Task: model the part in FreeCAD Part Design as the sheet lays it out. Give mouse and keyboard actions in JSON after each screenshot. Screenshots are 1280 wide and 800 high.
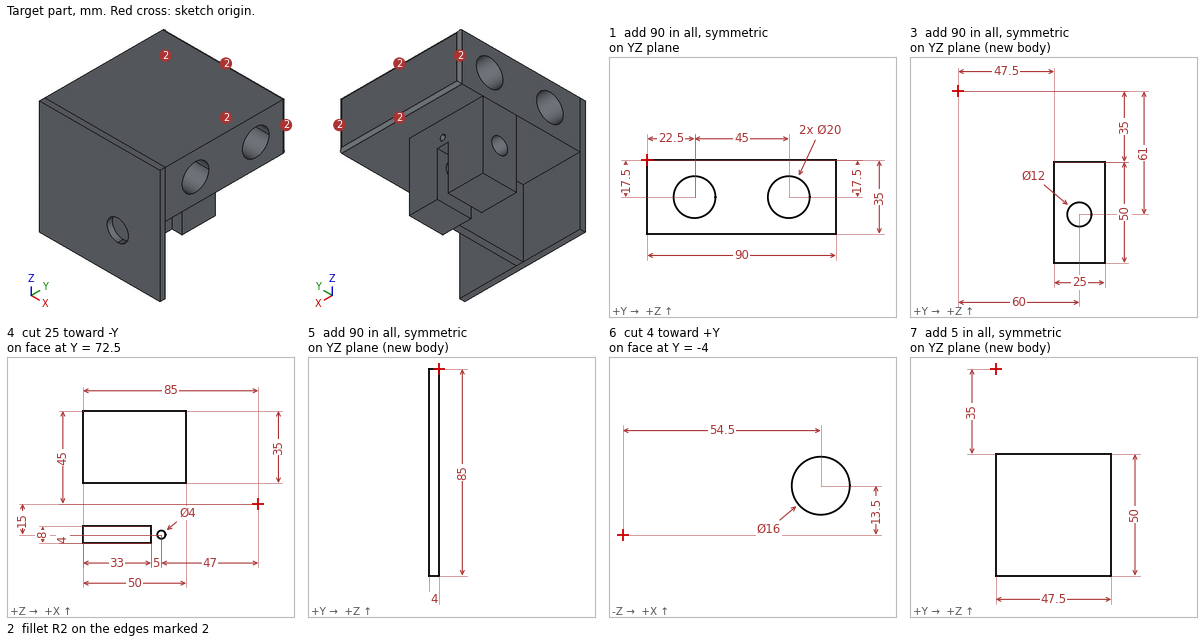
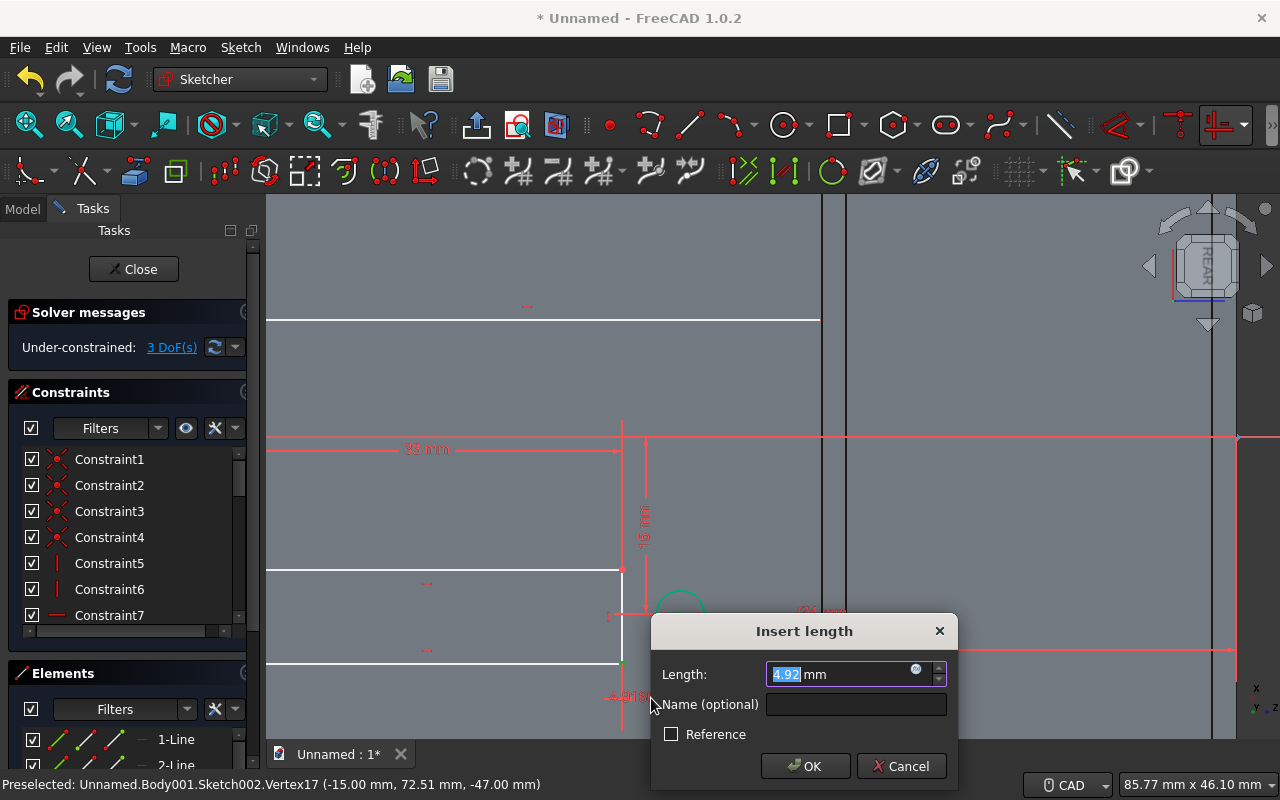
{"action": "type", "text": "5"}
{"action": "key", "text": "Return"}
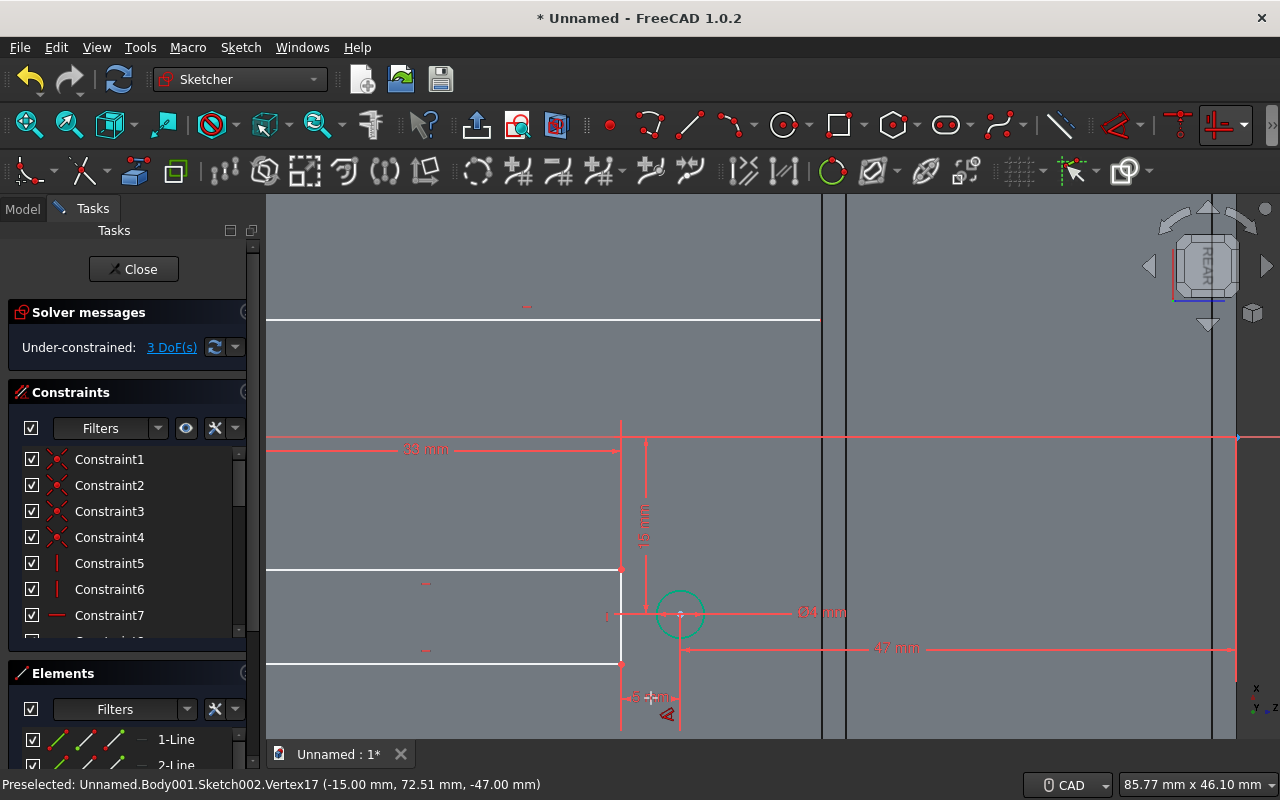
{"action": "left_click", "coordinate": [621, 664]}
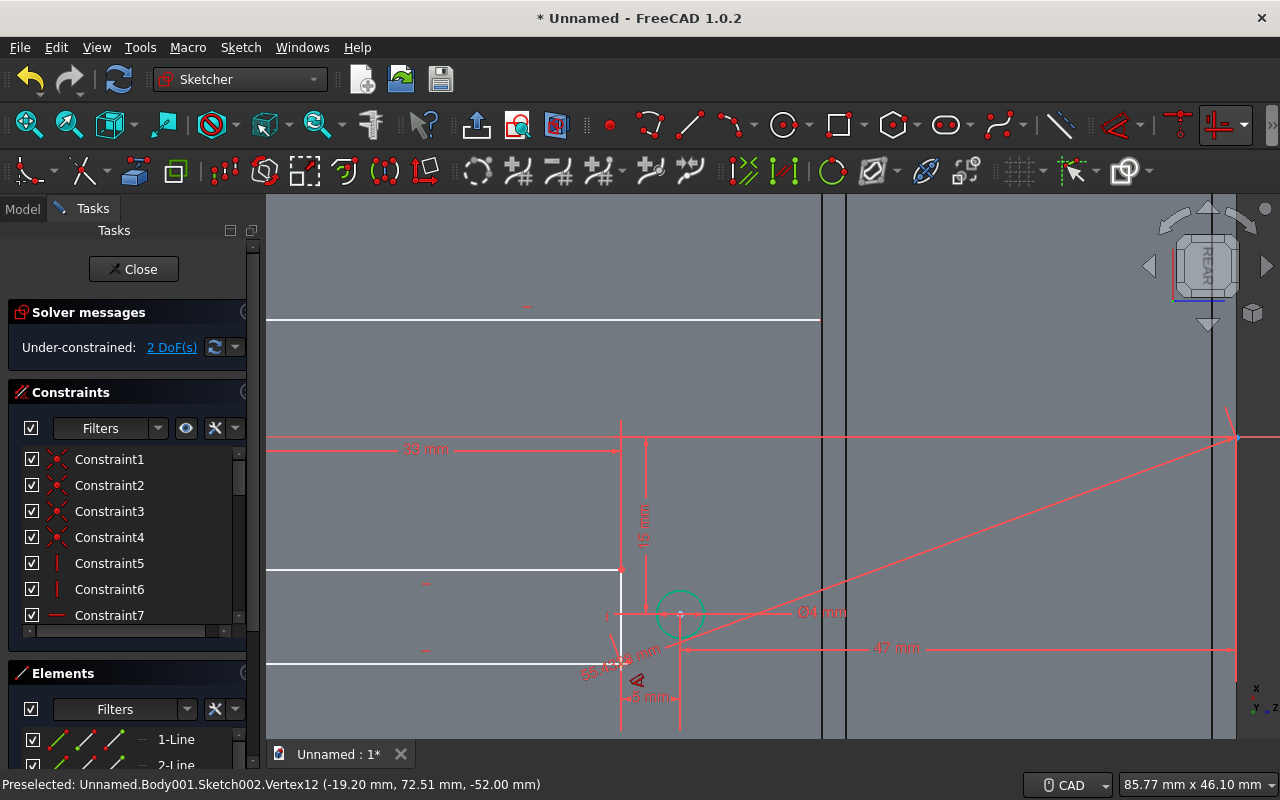
{"action": "left_click", "coordinate": [680, 614]}
{"action": "left_click", "coordinate": [587, 639]}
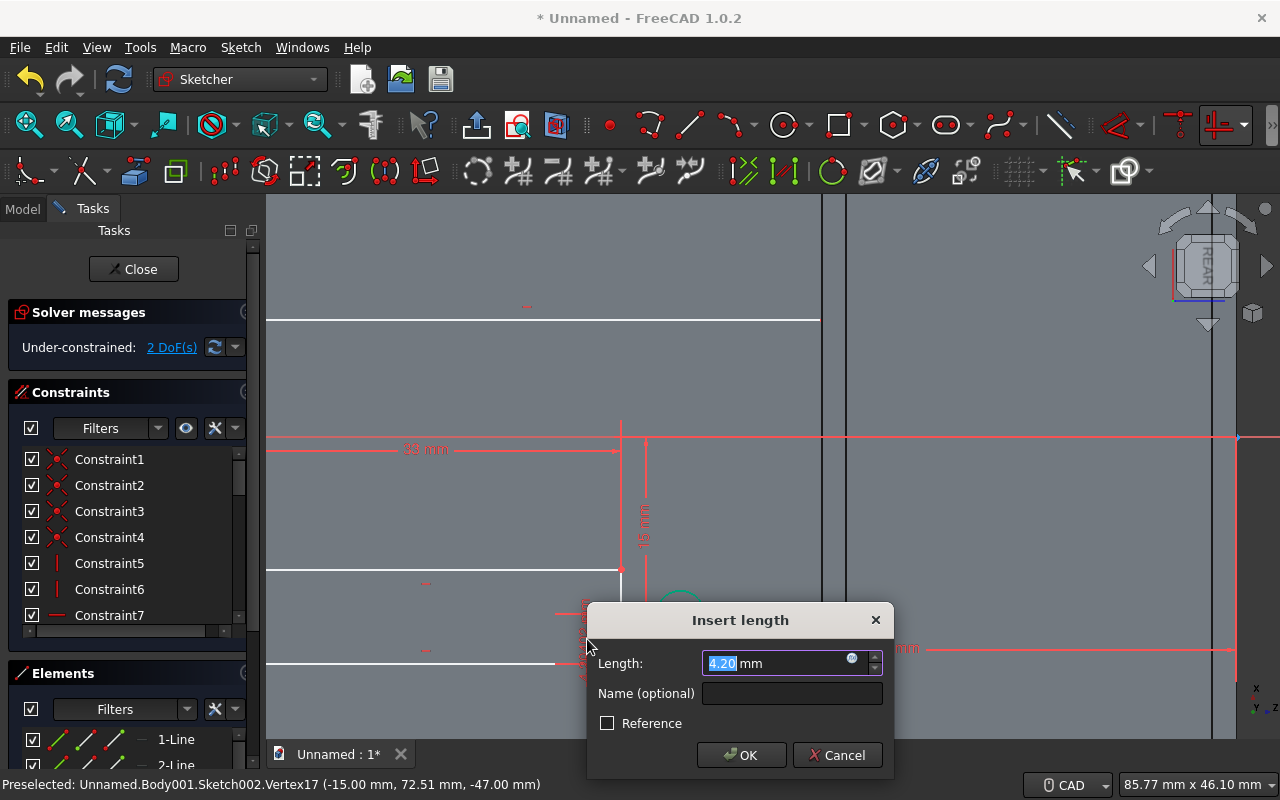
{"action": "type", "text": "4"}
{"action": "key", "text": "Return"}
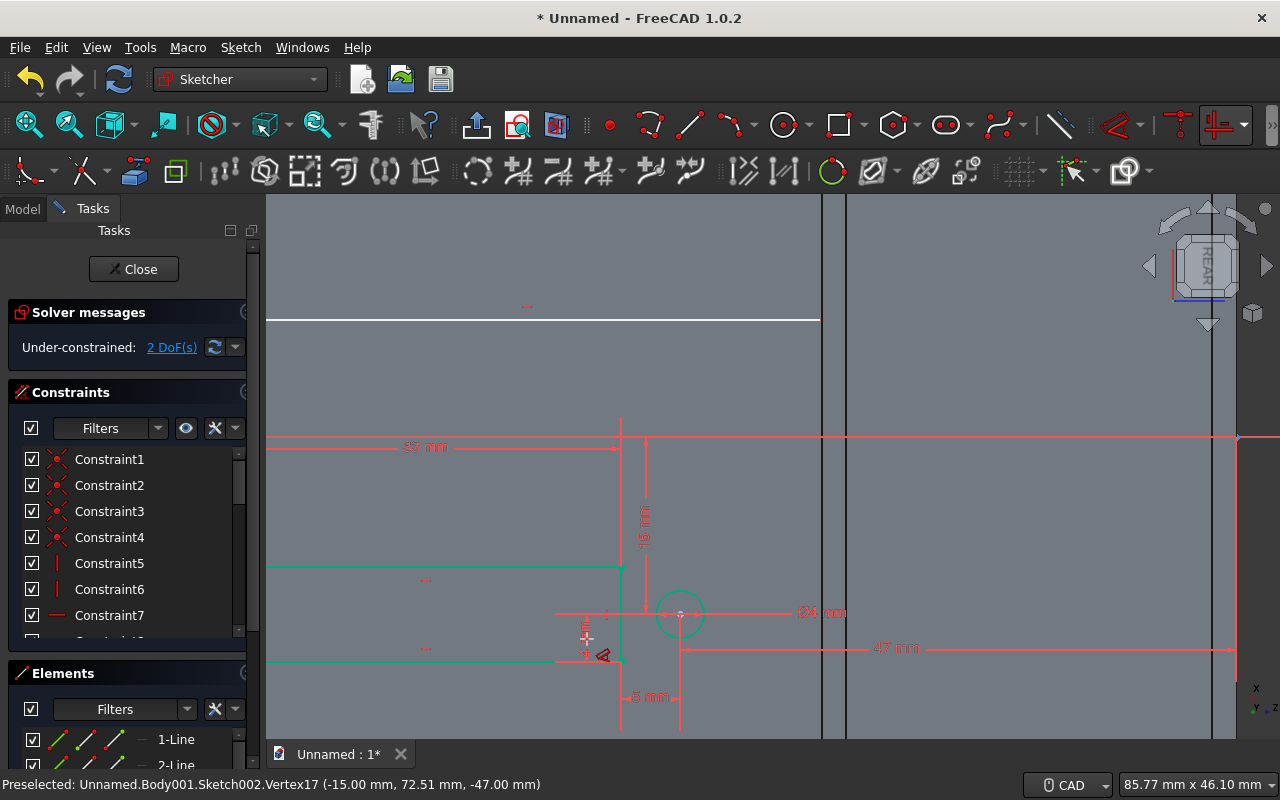
{"action": "scroll", "coordinate": [681, 616], "scroll_direction": "down", "scroll_amount": 4}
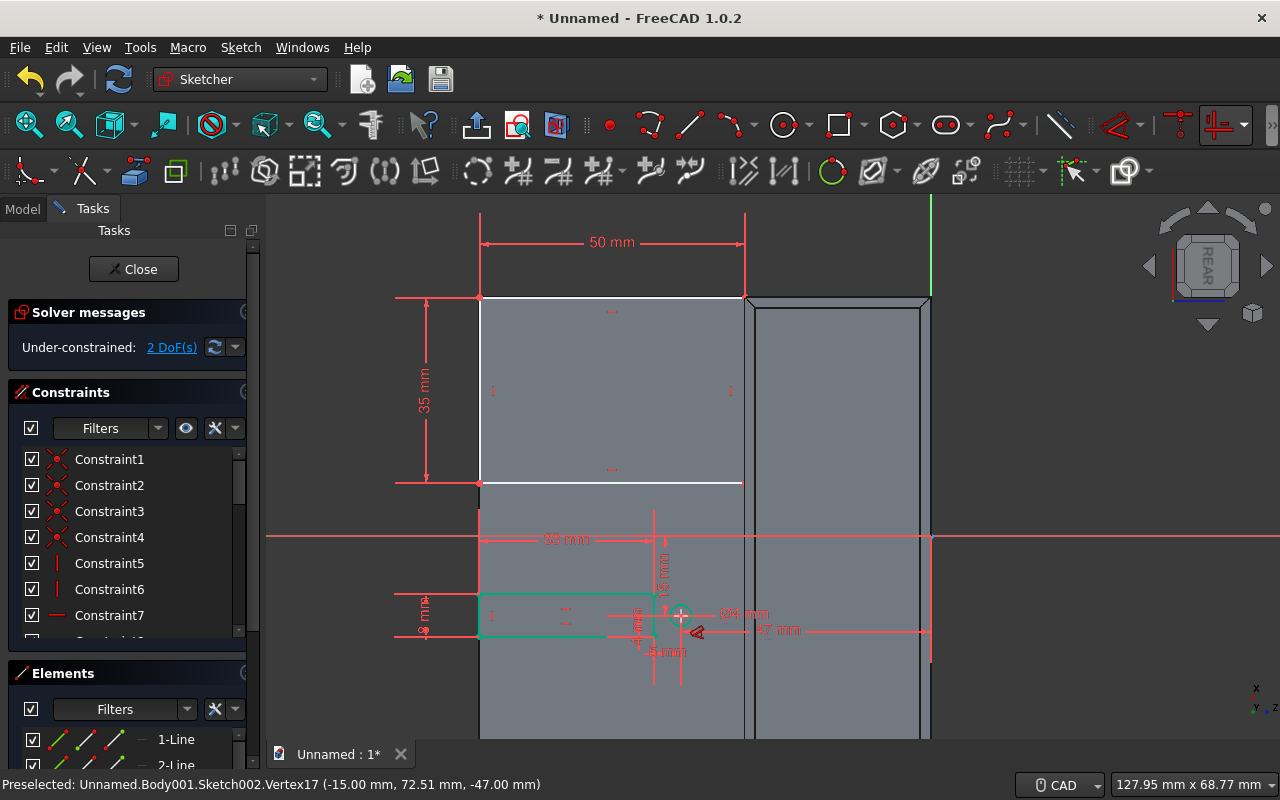
{"action": "left_click", "coordinate": [480, 298]}
{"action": "left_click", "coordinate": [705, 264]}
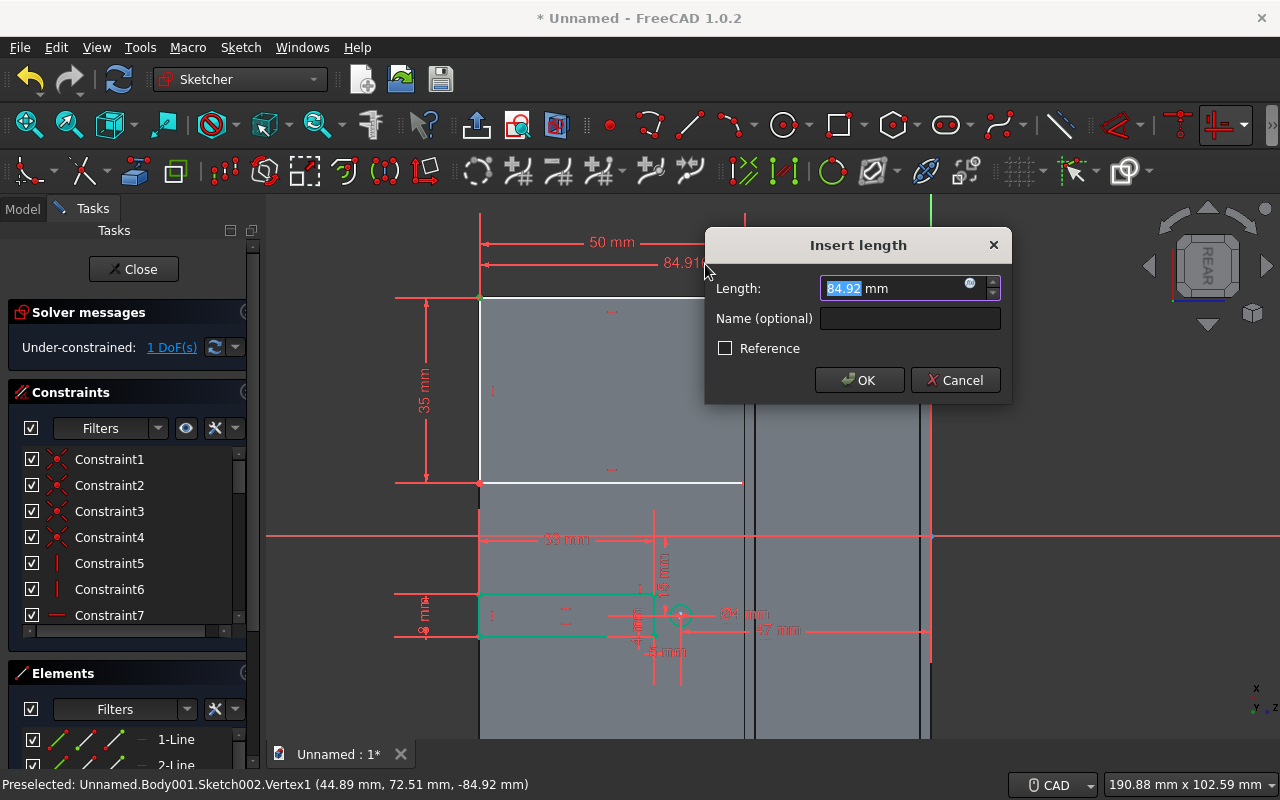
{"action": "type", "text": "85"}
{"action": "key", "text": "Return"}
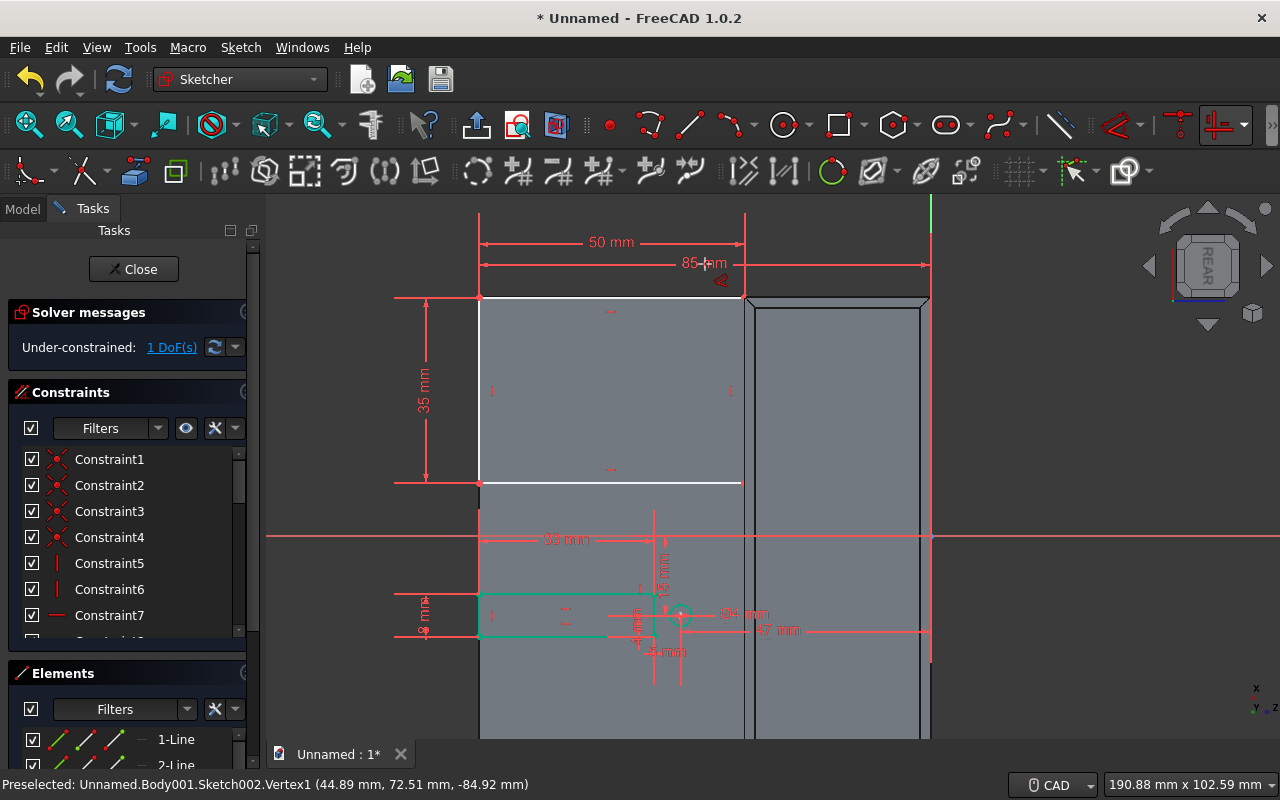
{"action": "left_click", "coordinate": [479, 298]}
{"action": "left_click", "coordinate": [965, 417]}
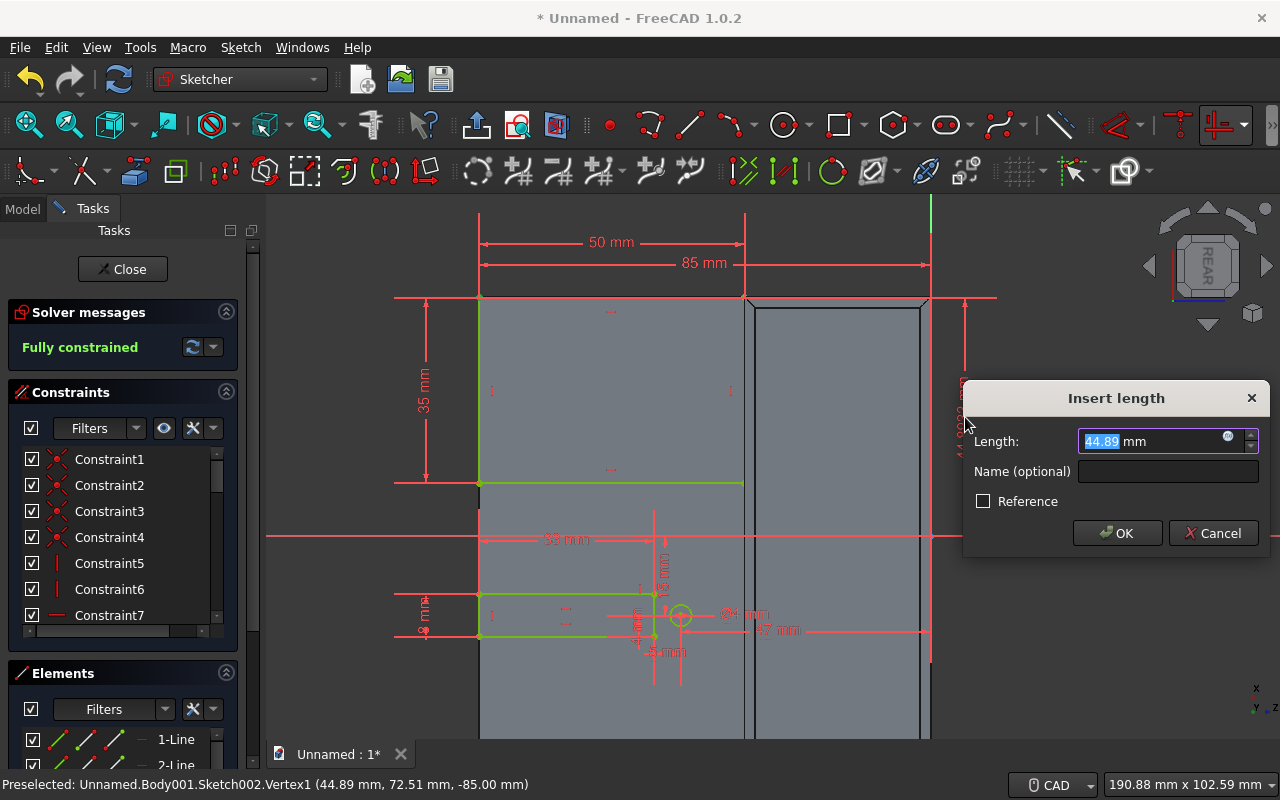
{"action": "type", "text": "45"}
{"action": "key", "text": "Return"}
{"action": "key", "text": "Escape"}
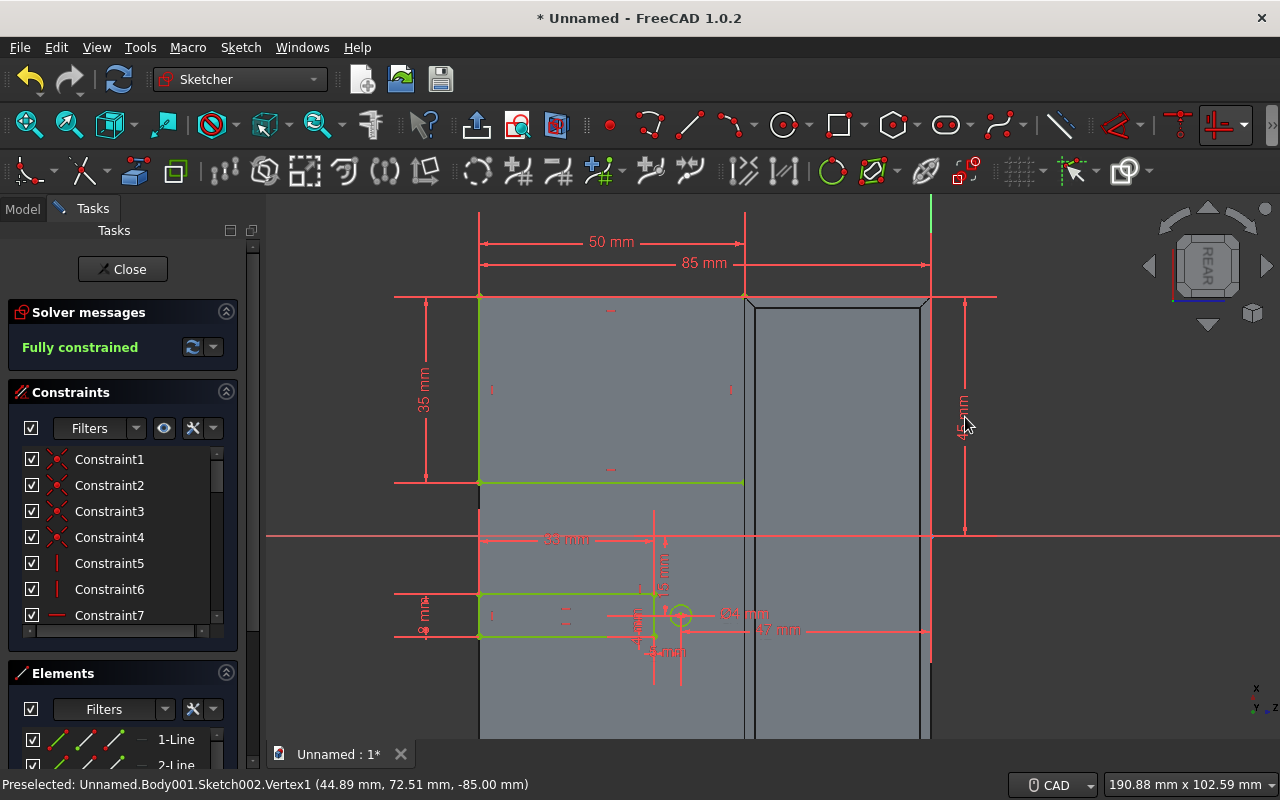
{"action": "left_click", "coordinate": [123, 269]}